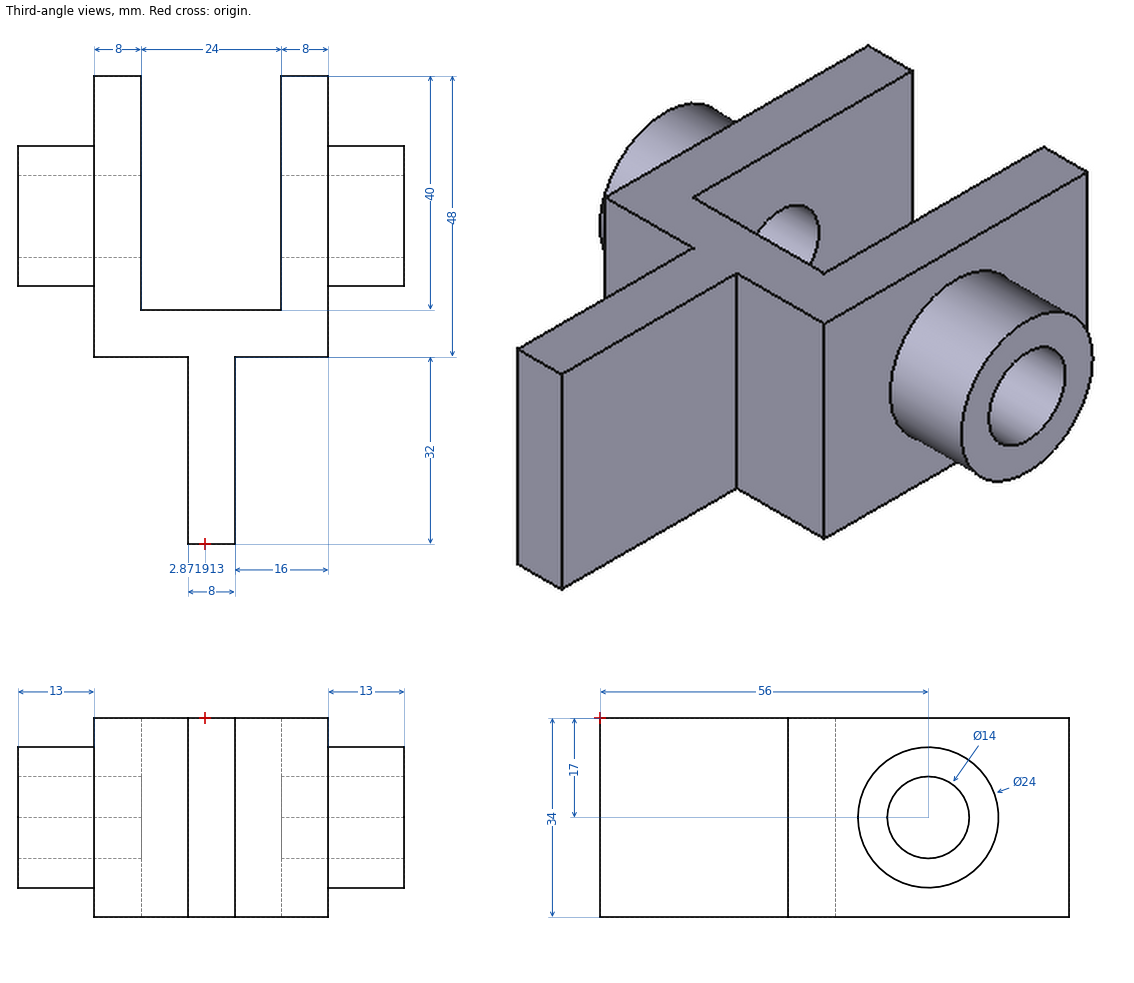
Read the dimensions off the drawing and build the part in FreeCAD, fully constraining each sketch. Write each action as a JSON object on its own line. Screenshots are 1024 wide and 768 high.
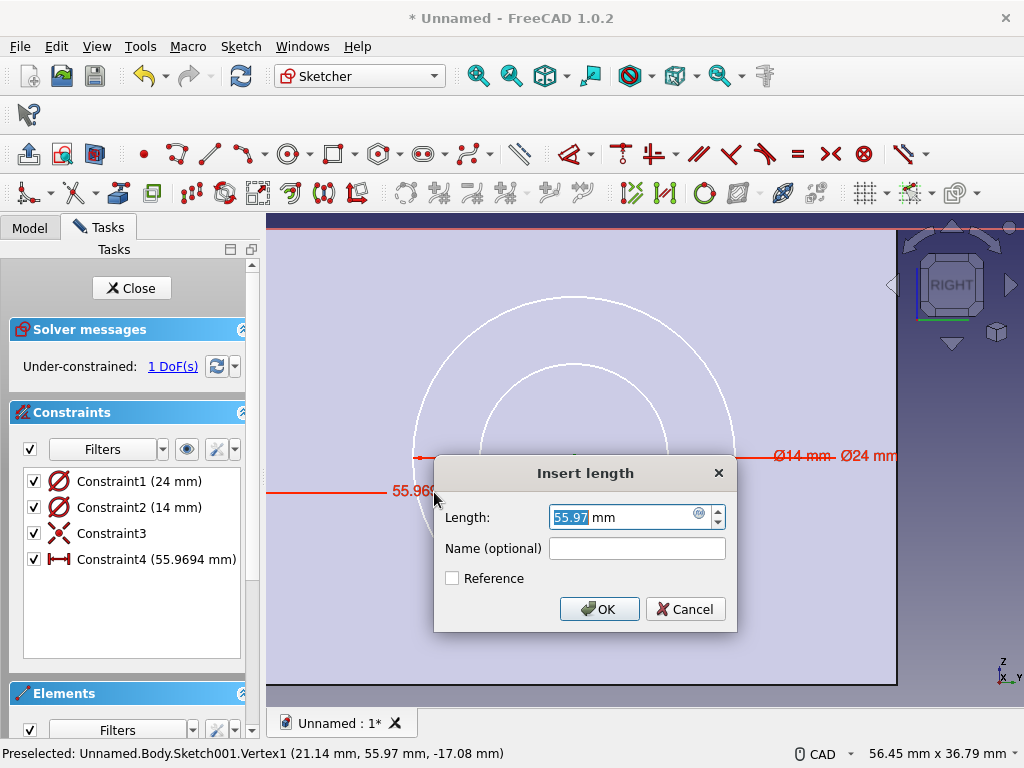
{"action": "type", "text": "56"}
{"action": "key", "text": "Return"}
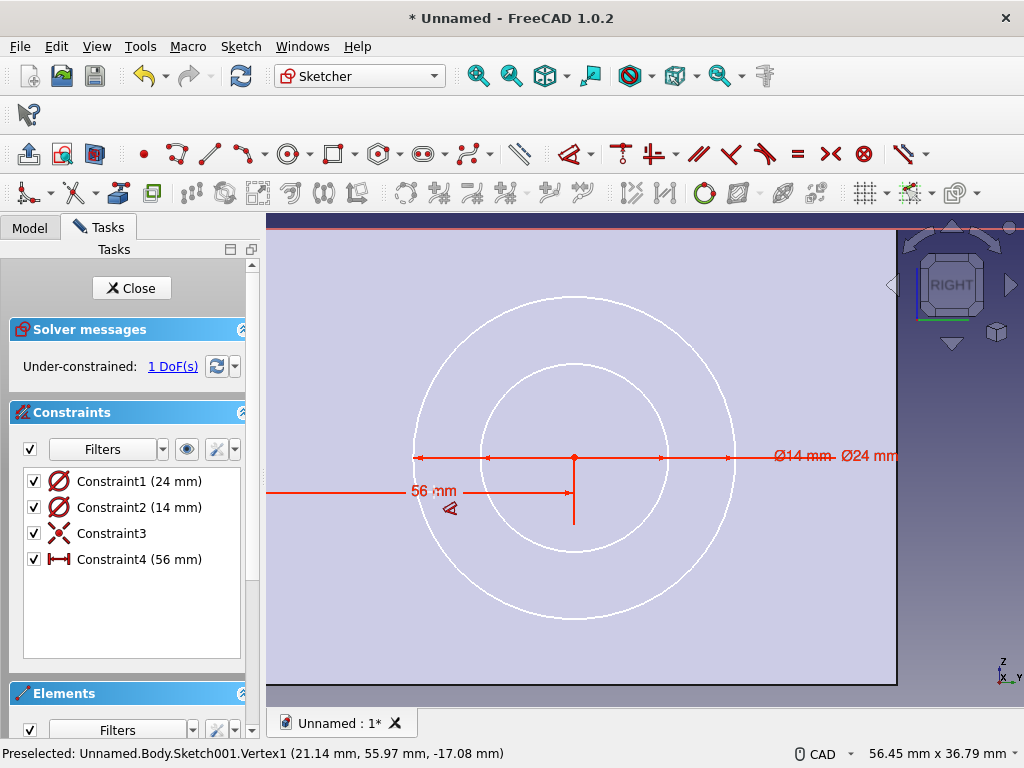
{"action": "left_click", "coordinate": [574, 458]}
{"action": "left_click", "coordinate": [608, 349]}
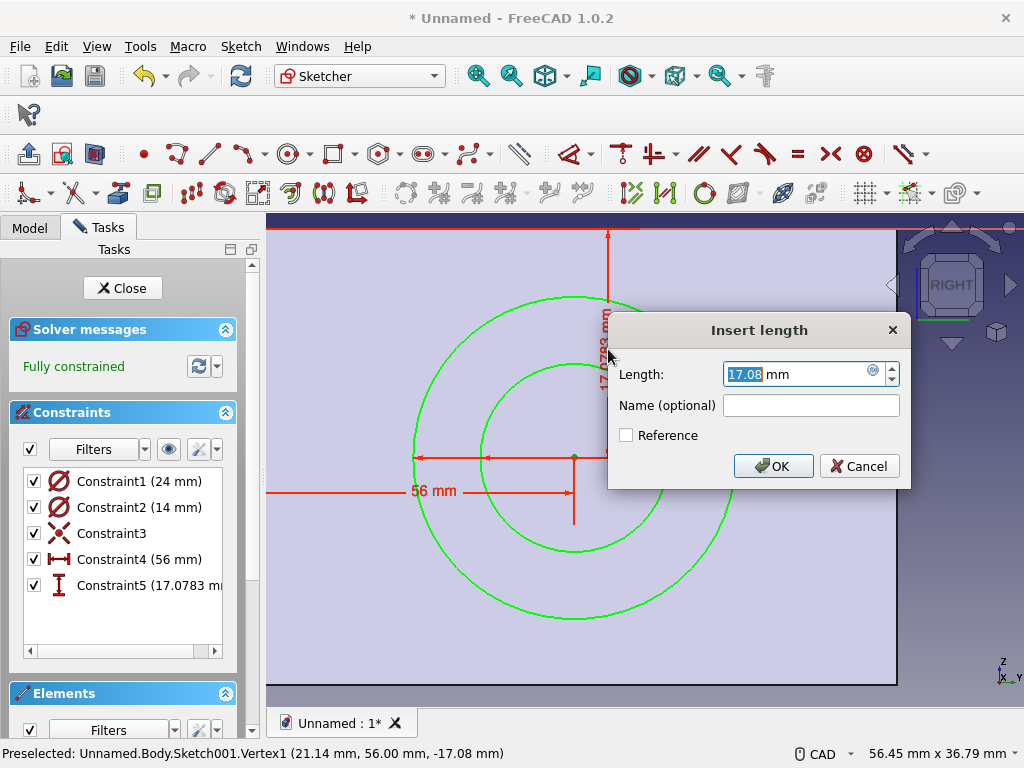
{"action": "type", "text": "17"}
{"action": "key", "text": "Return"}
{"action": "key", "text": "Escape"}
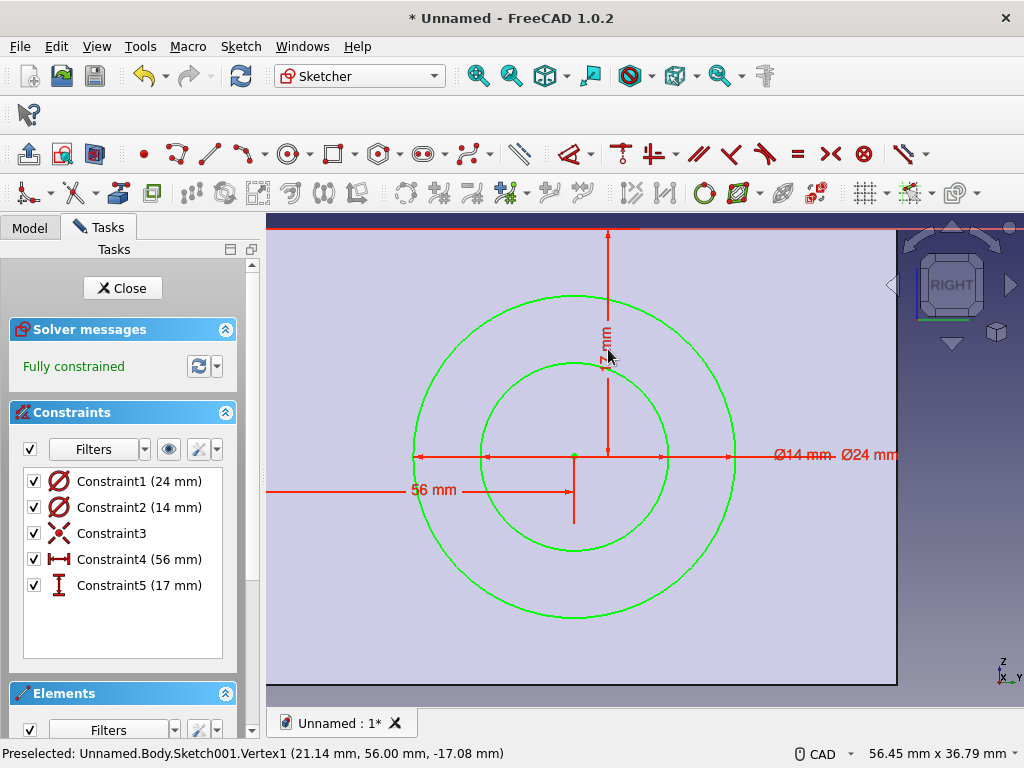
{"action": "left_click", "coordinate": [123, 288]}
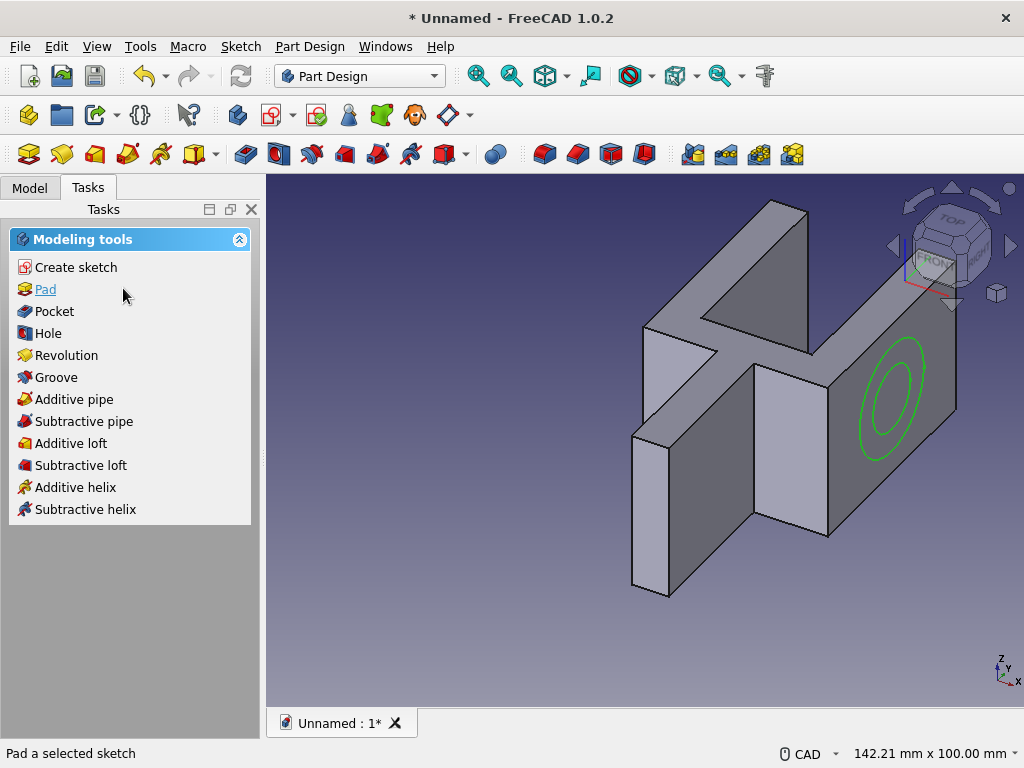
{"action": "left_click", "coordinate": [29, 154]}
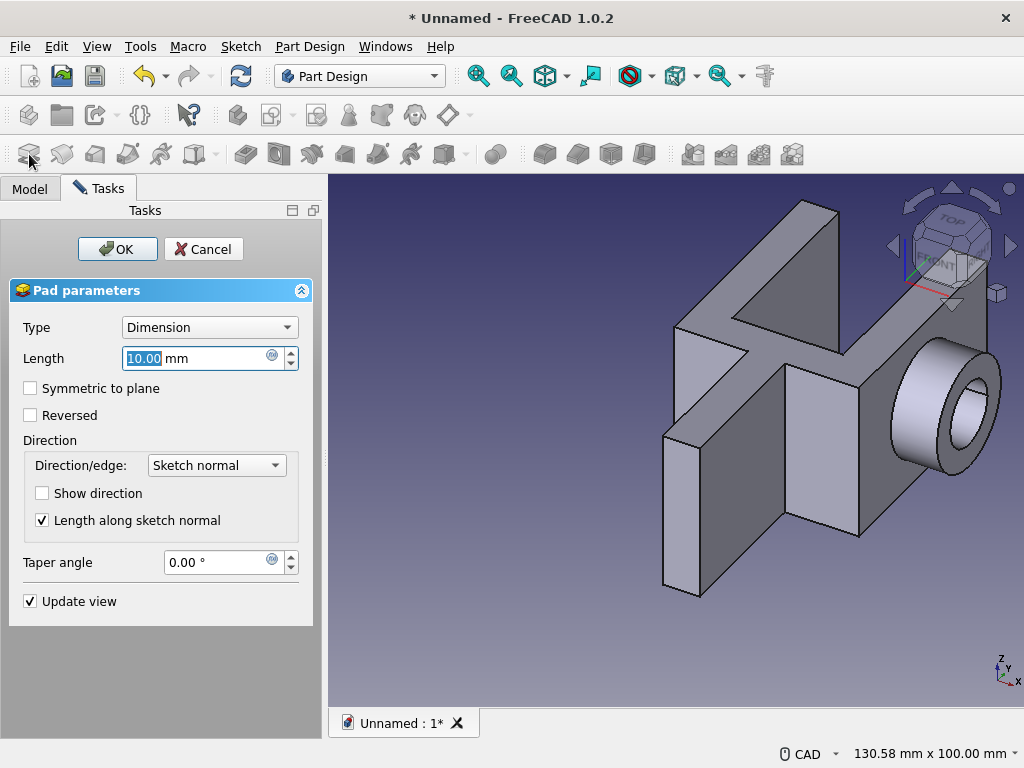
{"action": "type", "text": "13"}
{"action": "key", "text": "Tab"}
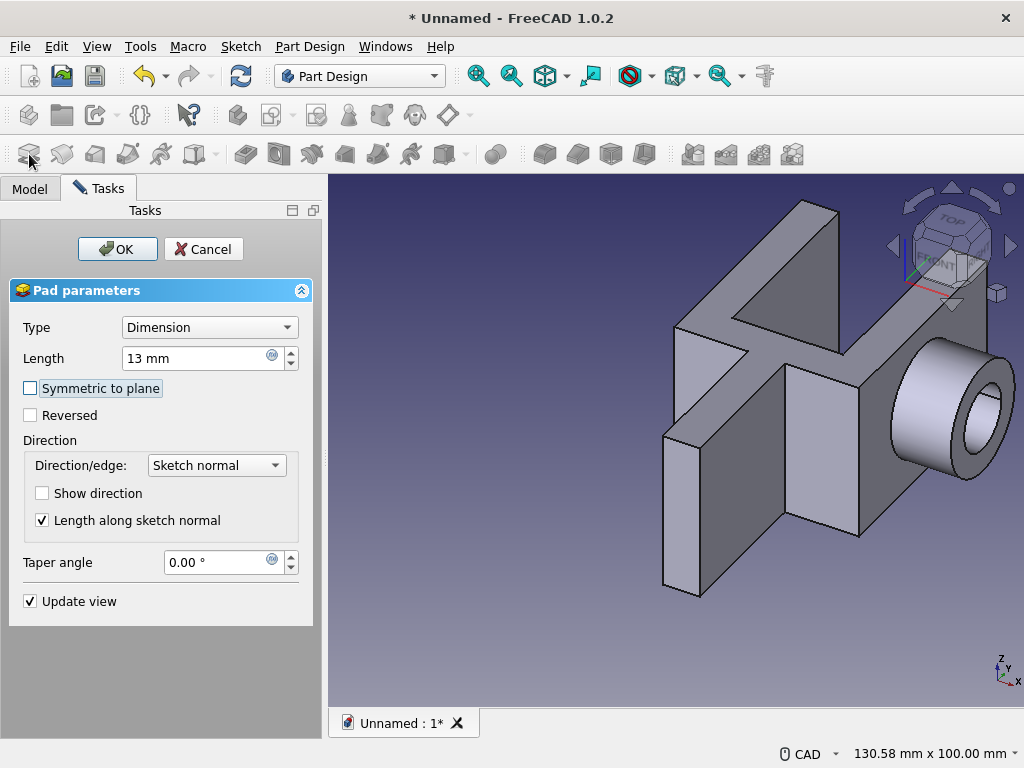
{"action": "left_click", "coordinate": [118, 249]}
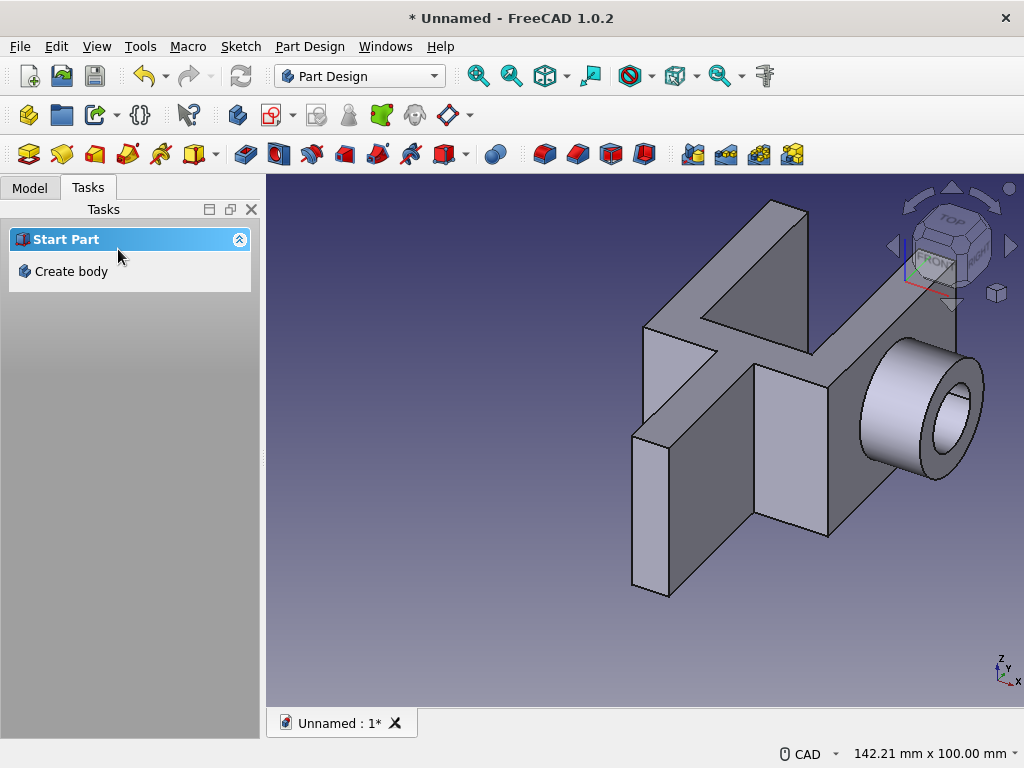
{"action": "left_click", "coordinate": [30, 188]}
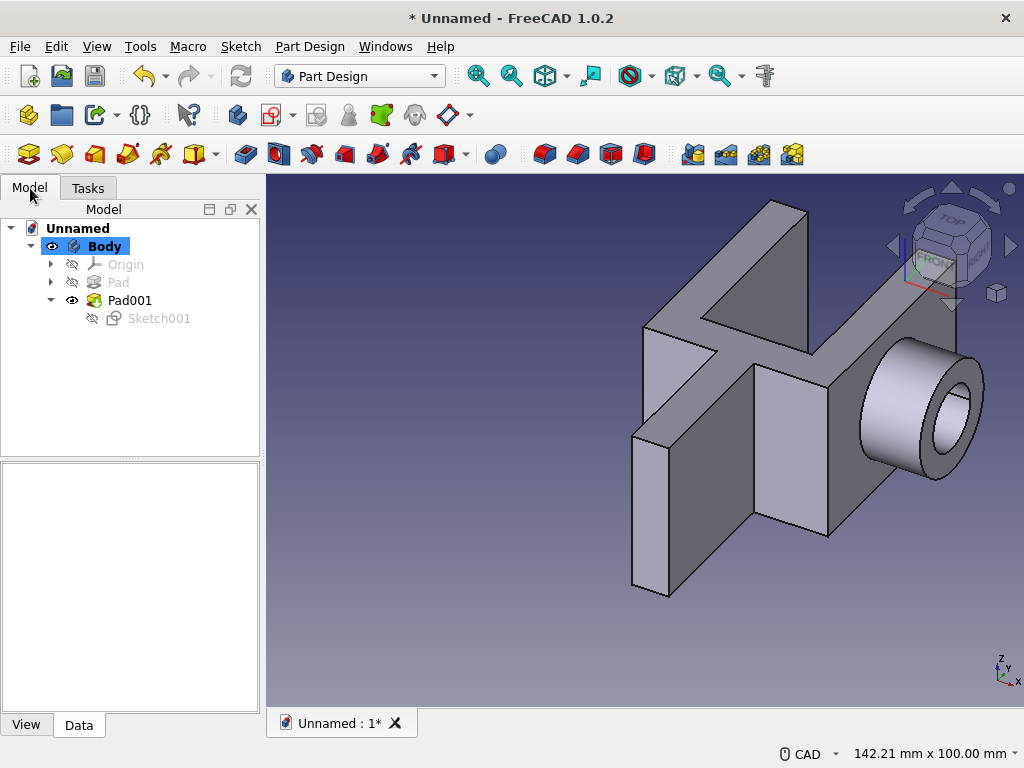
{"action": "left_click", "coordinate": [51, 264]}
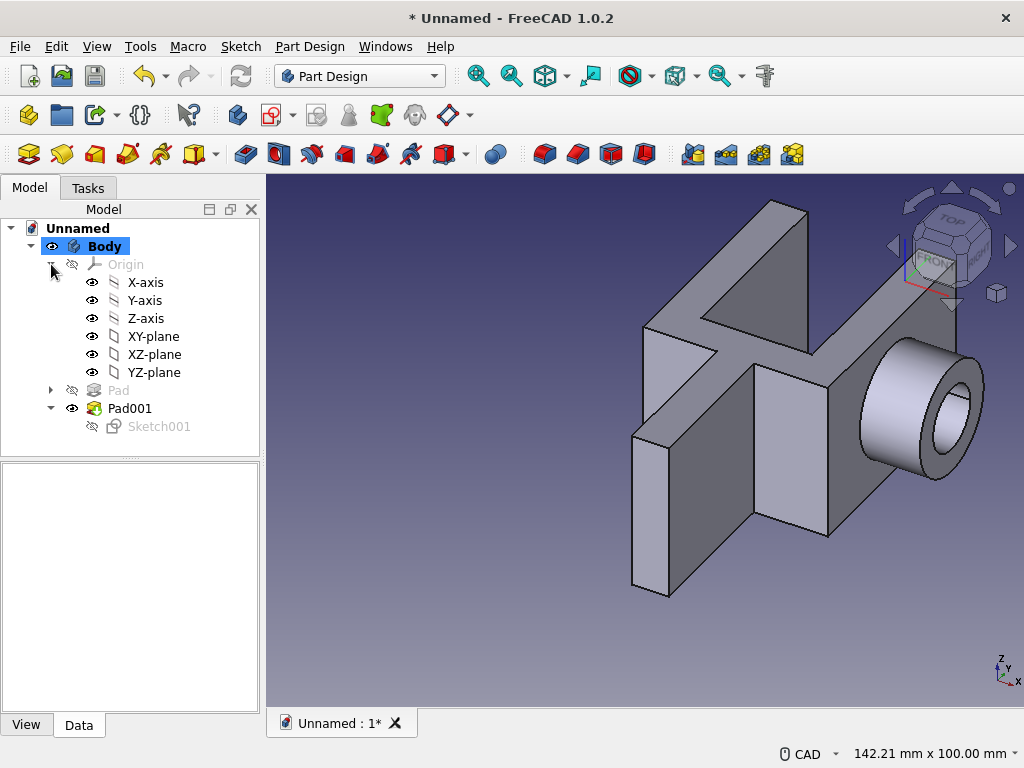
{"action": "left_click", "coordinate": [137, 372]}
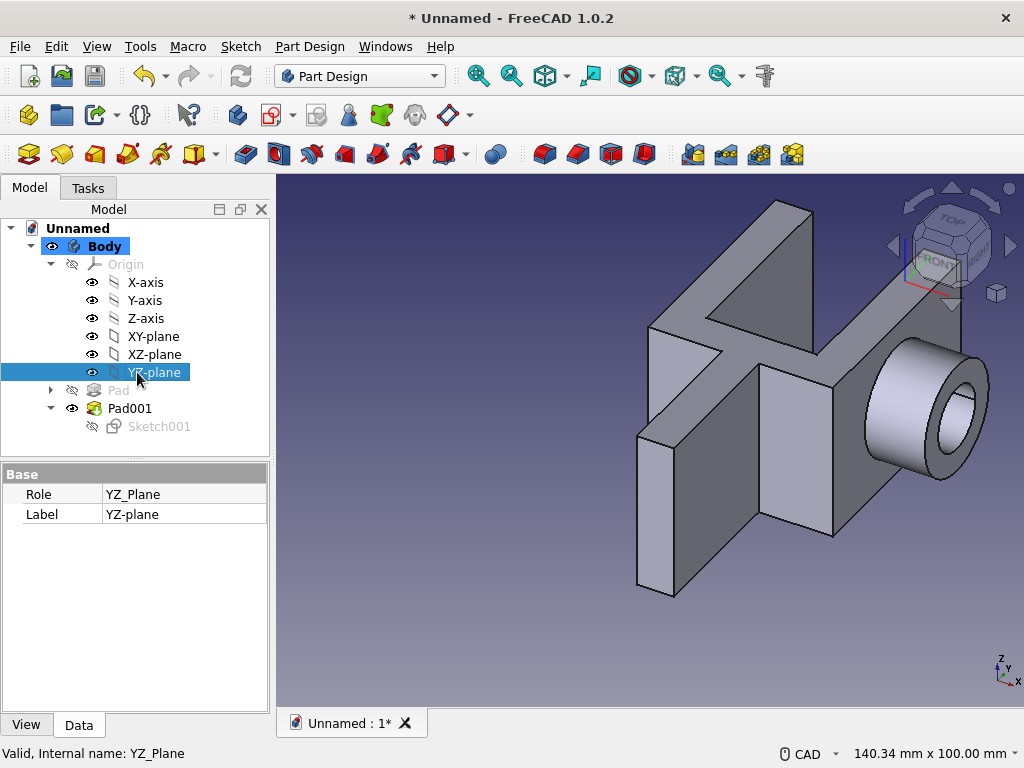
{"action": "left_click", "coordinate": [448, 116]}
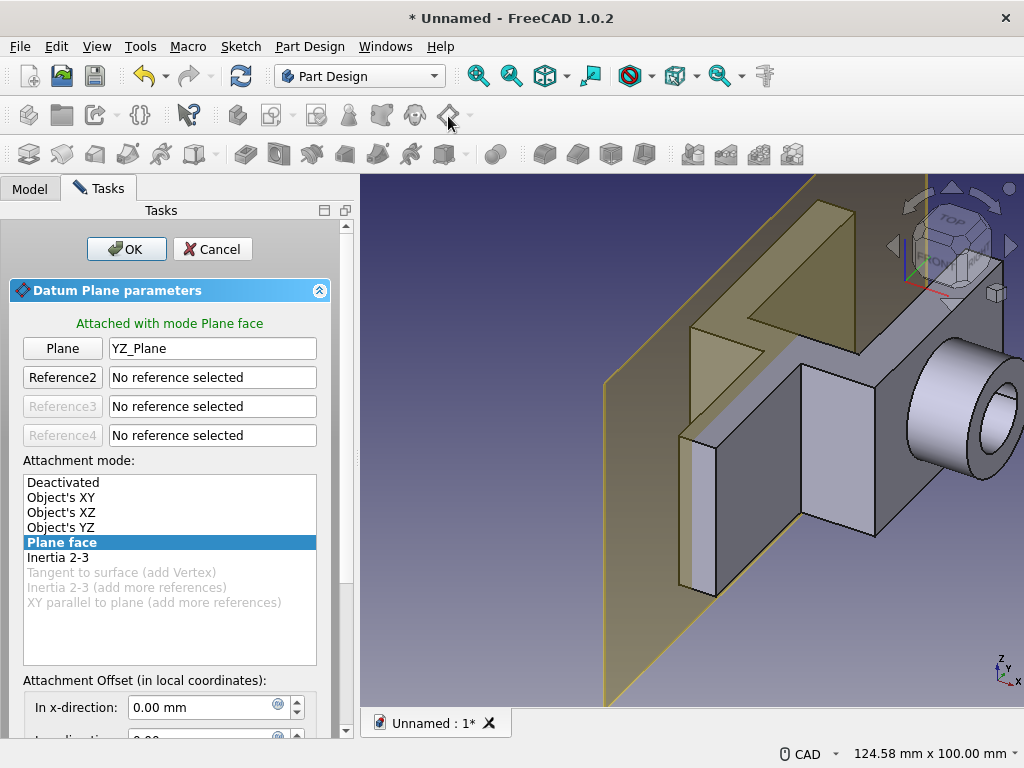
{"action": "scroll", "coordinate": [346, 479], "scroll_direction": "down", "scroll_amount": 2}